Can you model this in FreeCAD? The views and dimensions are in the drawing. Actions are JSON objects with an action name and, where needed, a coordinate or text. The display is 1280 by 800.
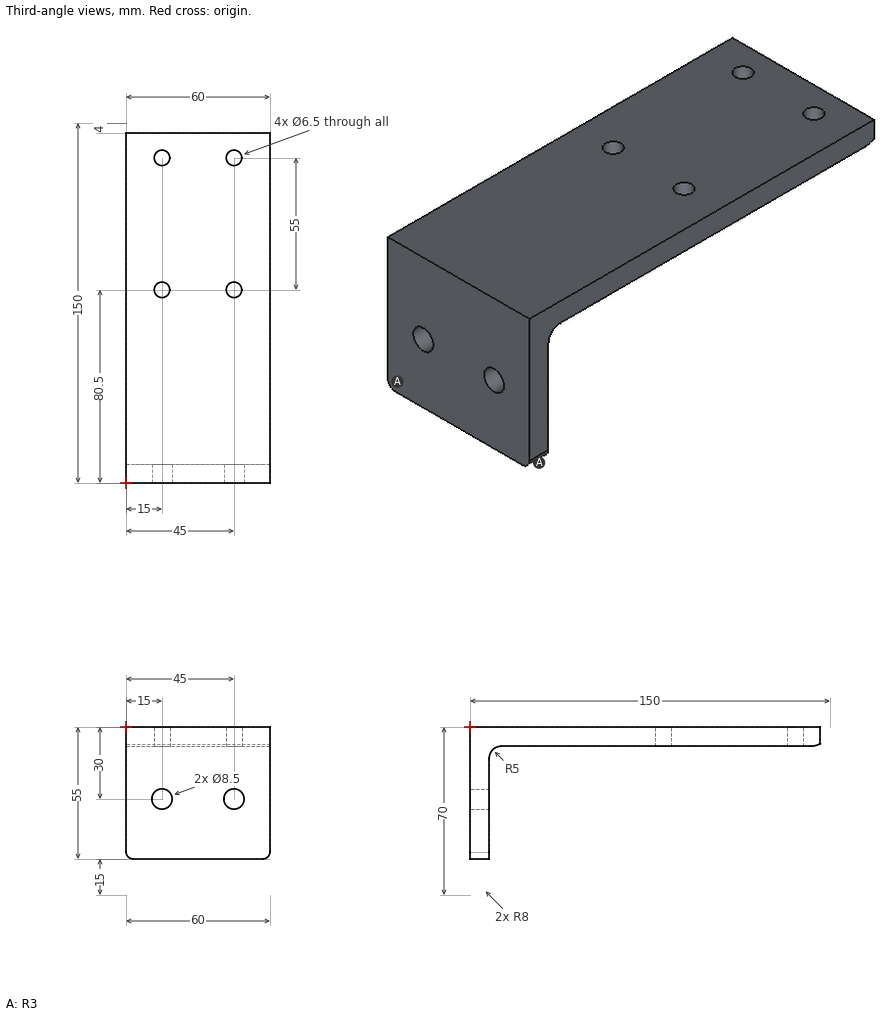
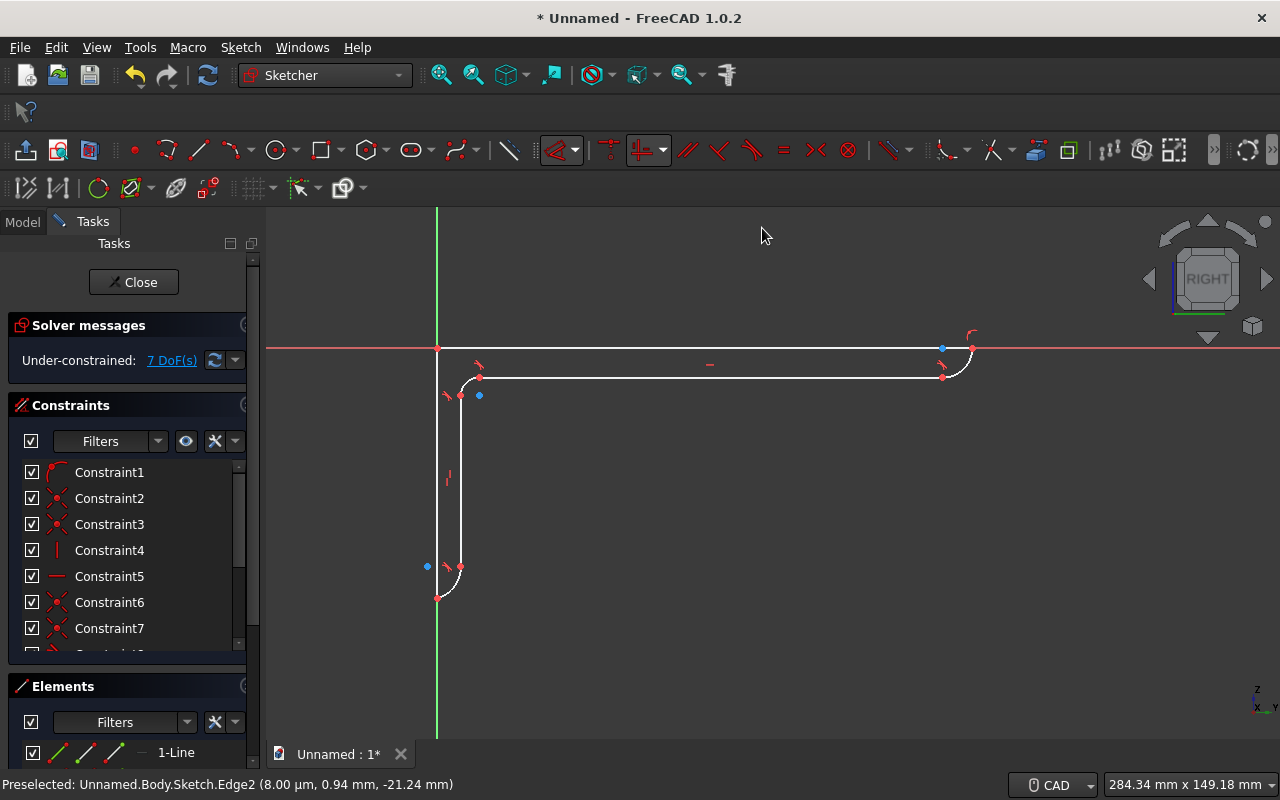
{"action": "scroll", "coordinate": [448, 593], "scroll_direction": "up", "scroll_amount": 2}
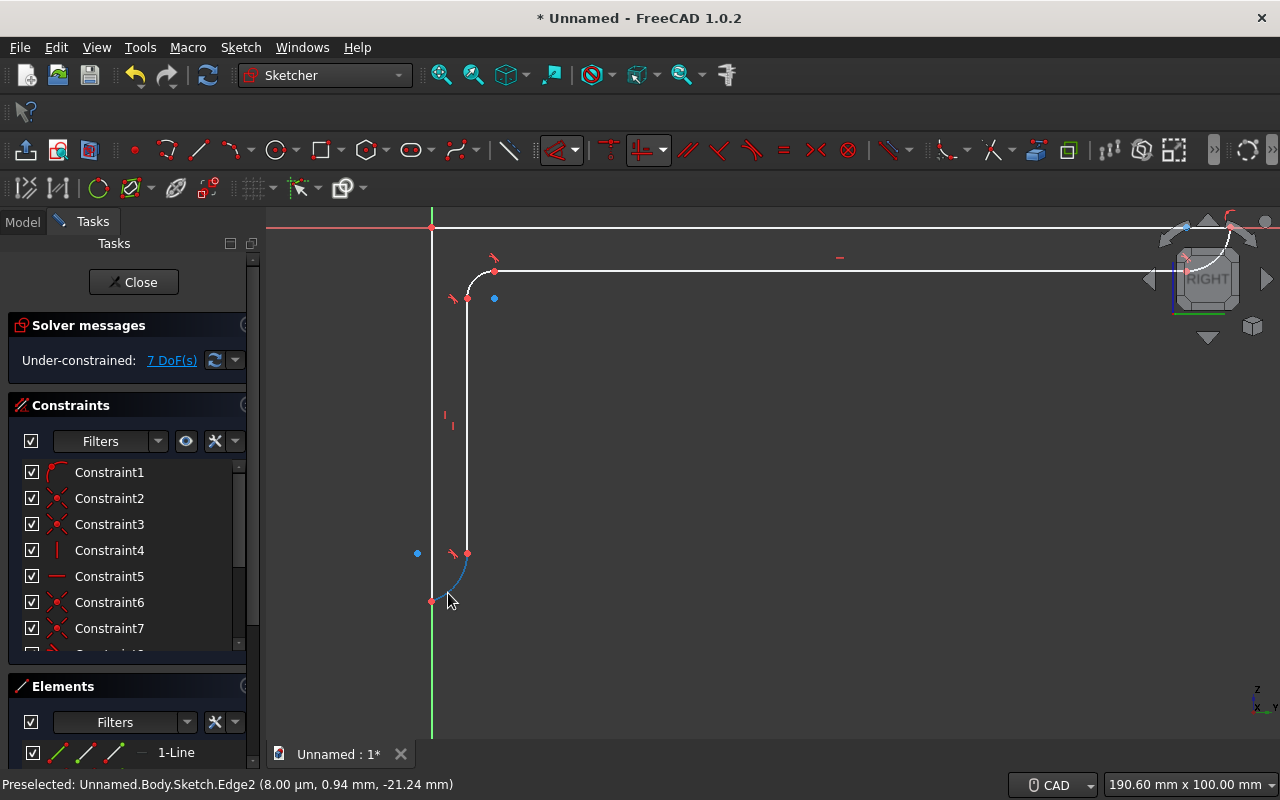
{"action": "left_click", "coordinate": [449, 592]}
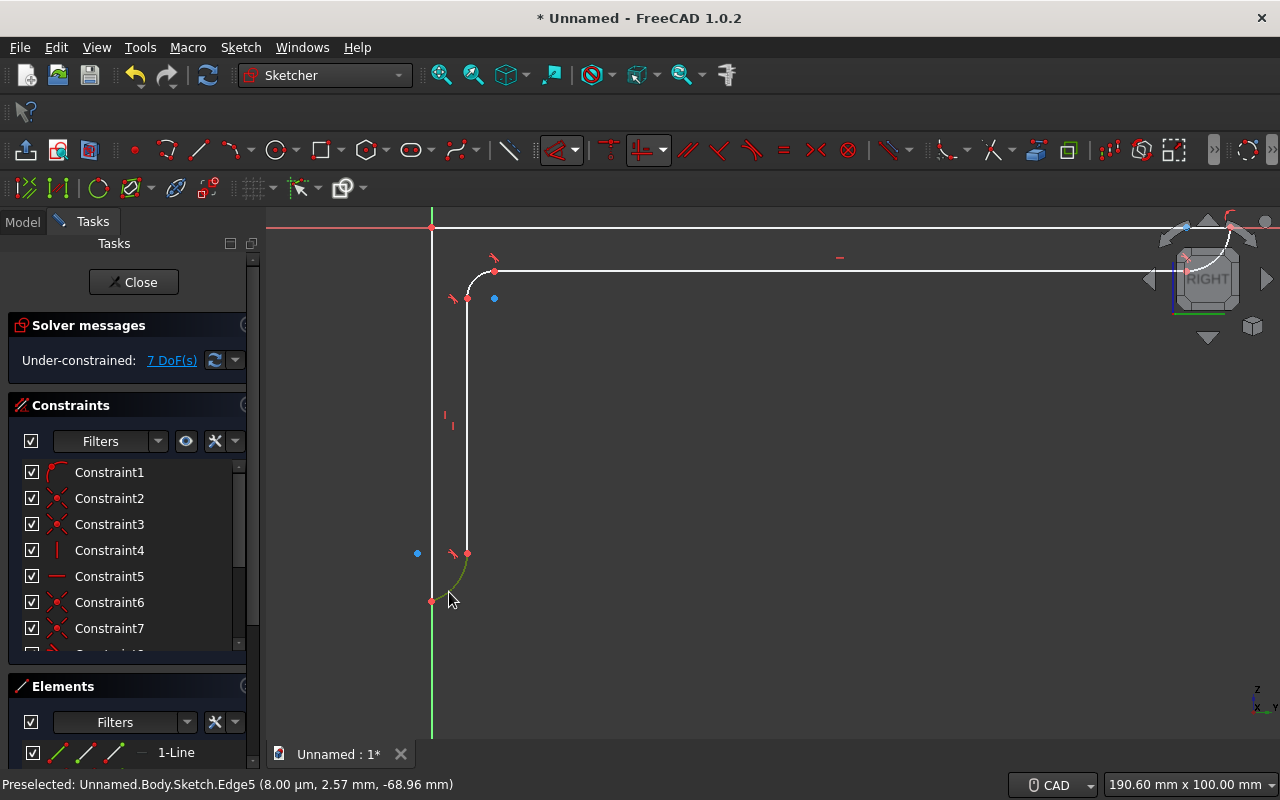
{"action": "scroll", "coordinate": [448, 593], "scroll_direction": "down", "scroll_amount": 2}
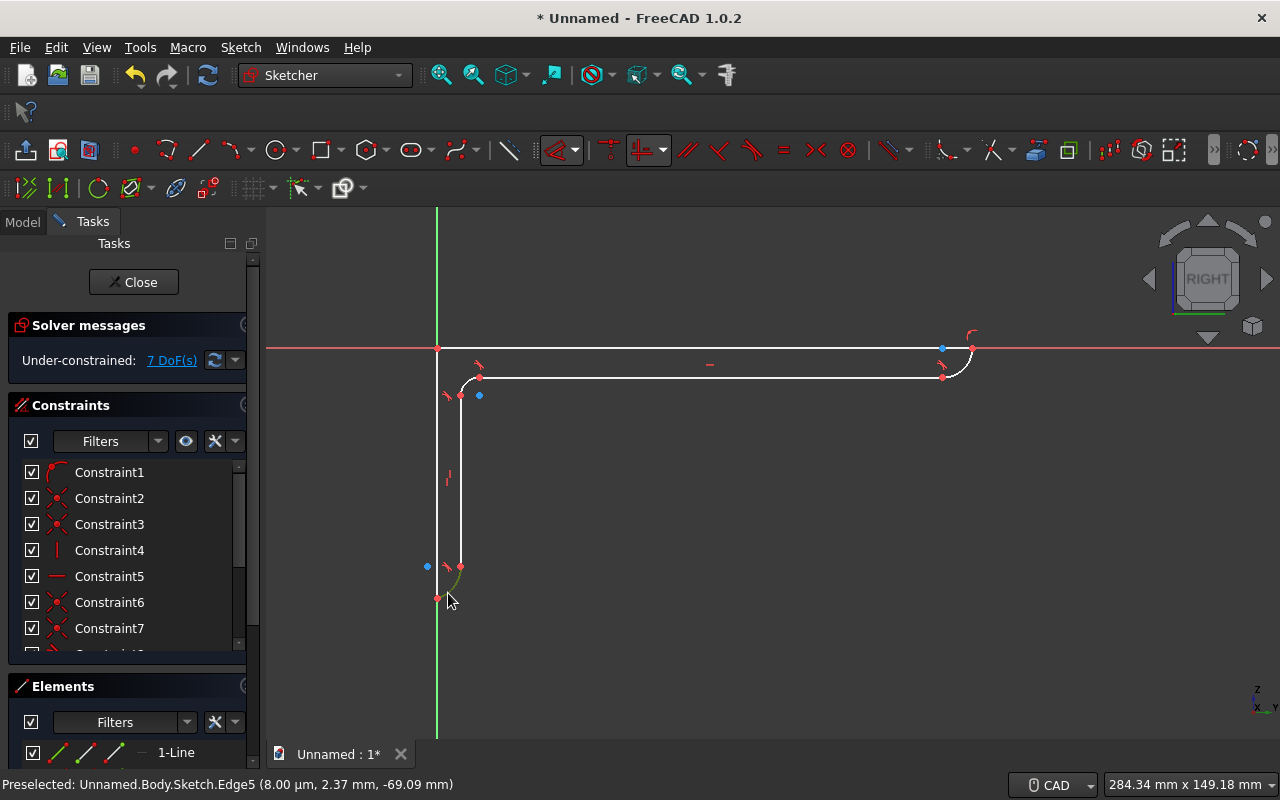
{"action": "left_click", "coordinate": [956, 374]}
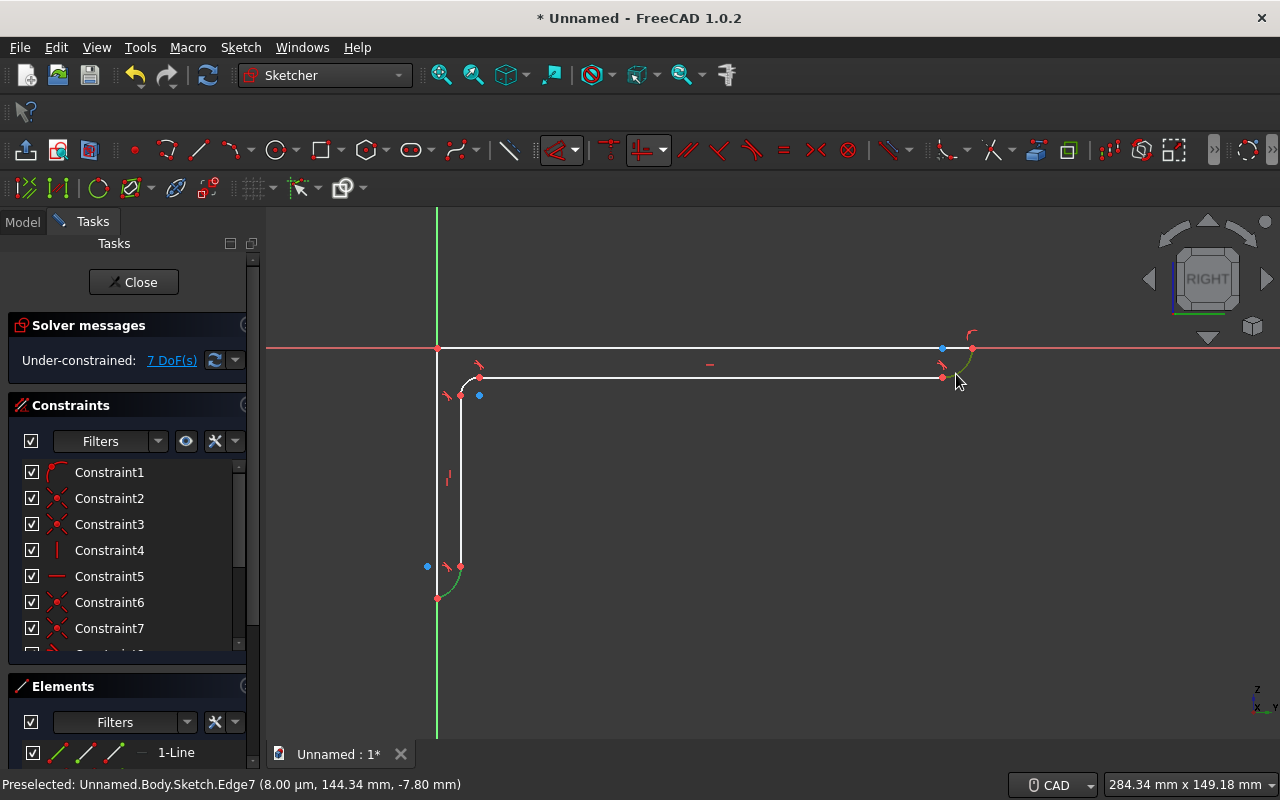
{"action": "key", "text": "e"}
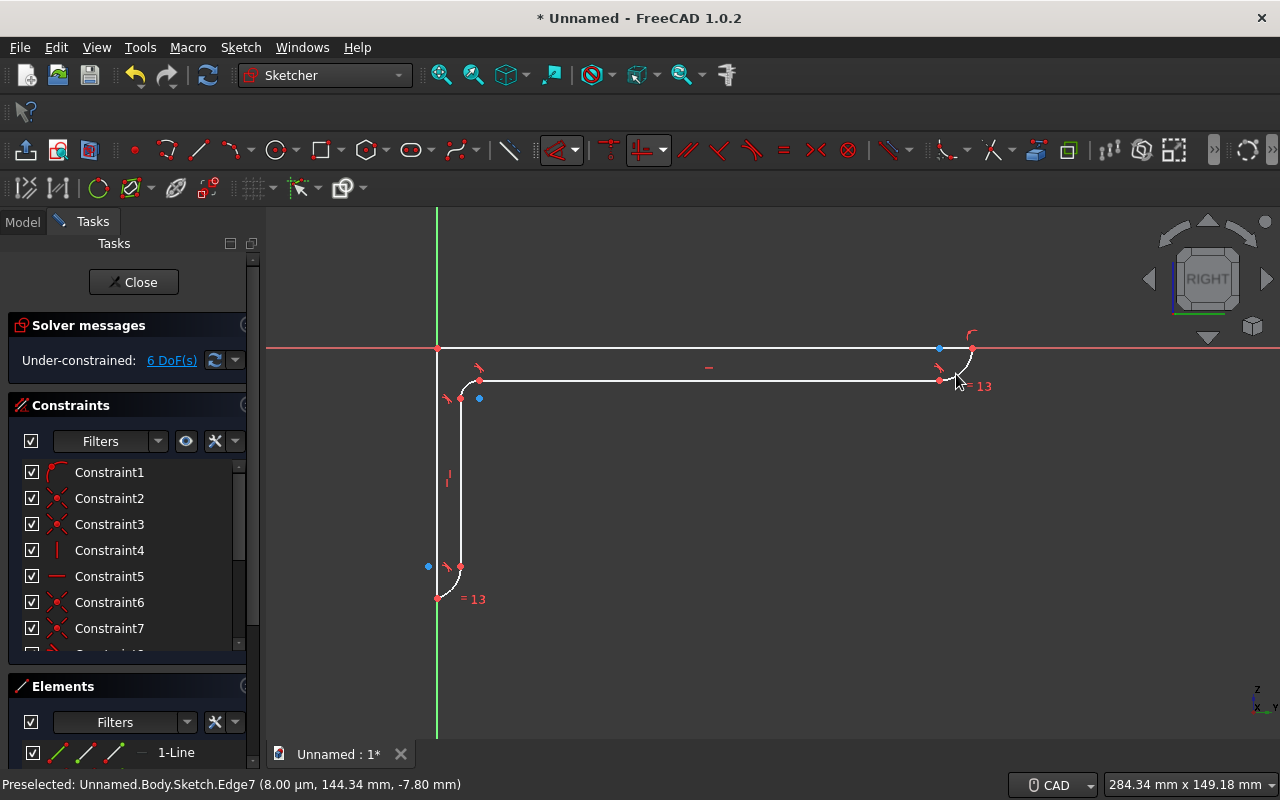
{"action": "left_click", "coordinate": [428, 567]}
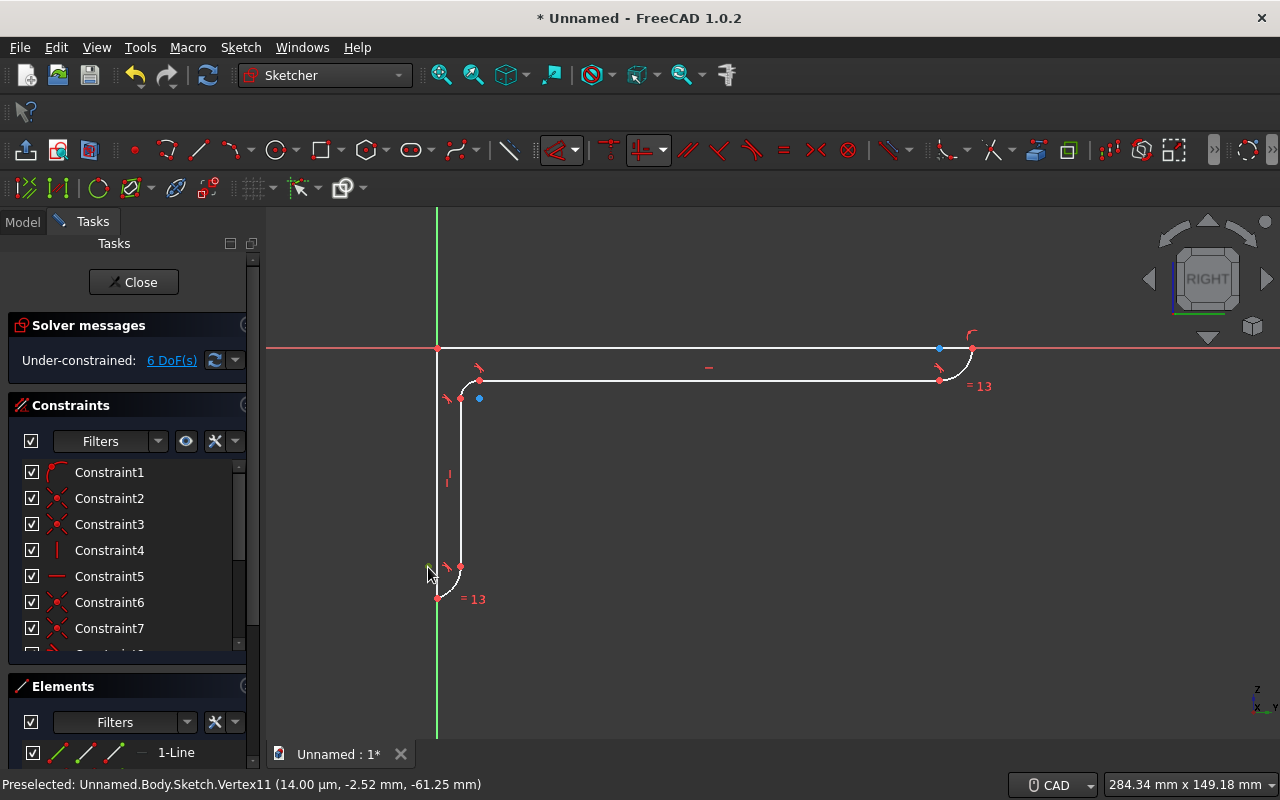
{"action": "left_click", "coordinate": [437, 677]}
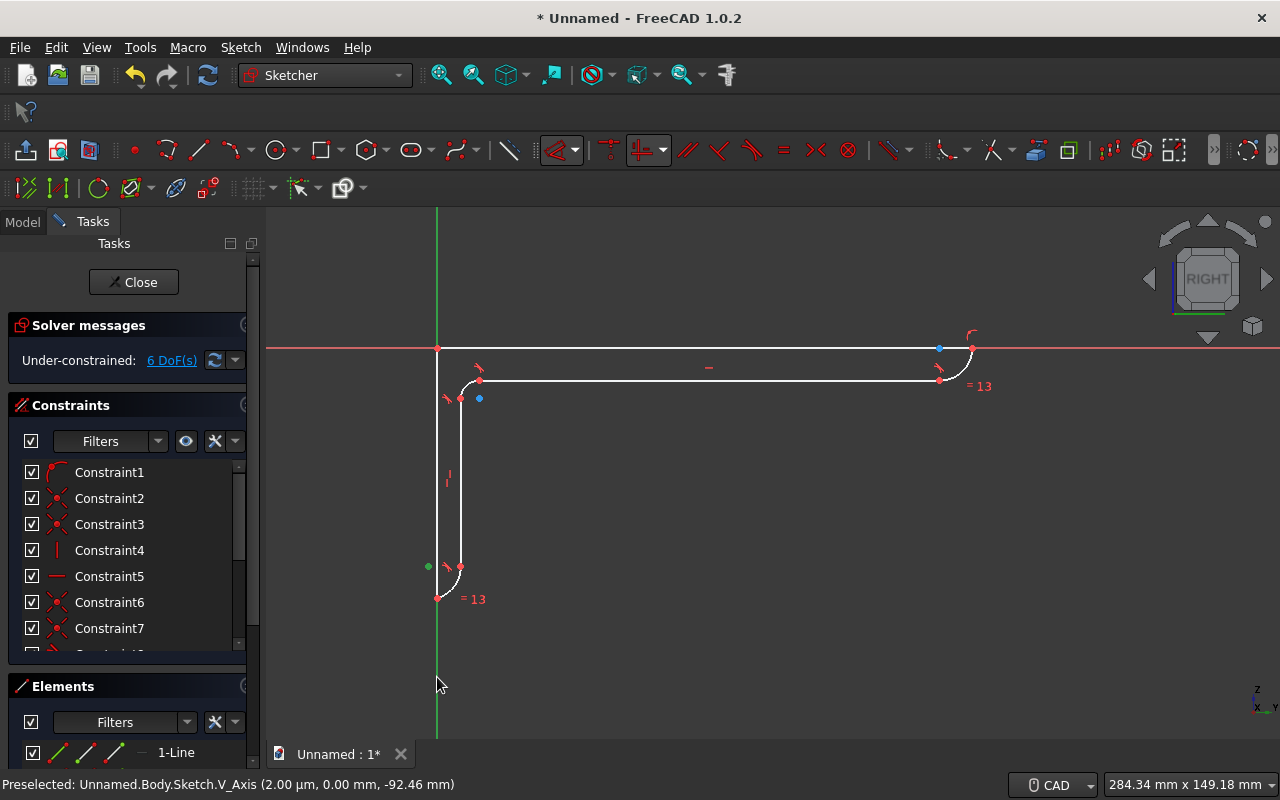
{"action": "key", "text": "c"}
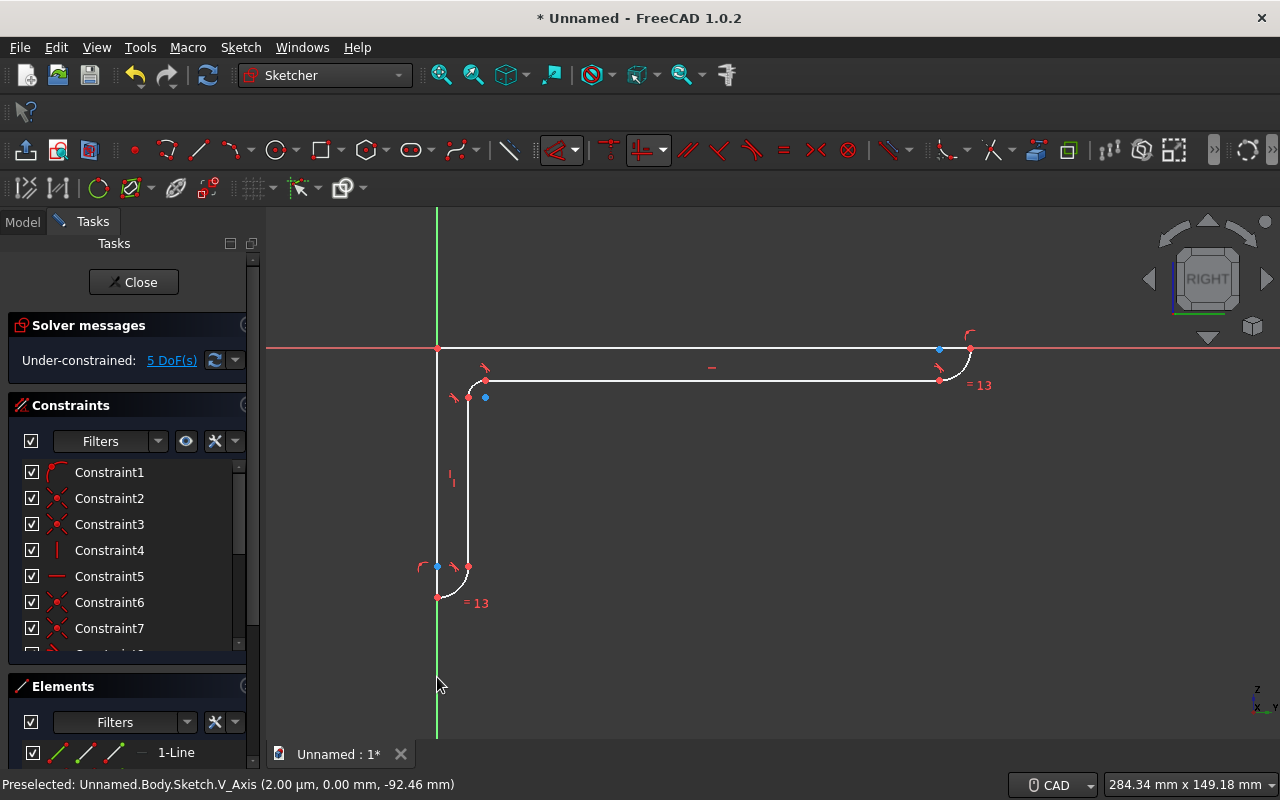
{"action": "left_click", "coordinate": [940, 350]}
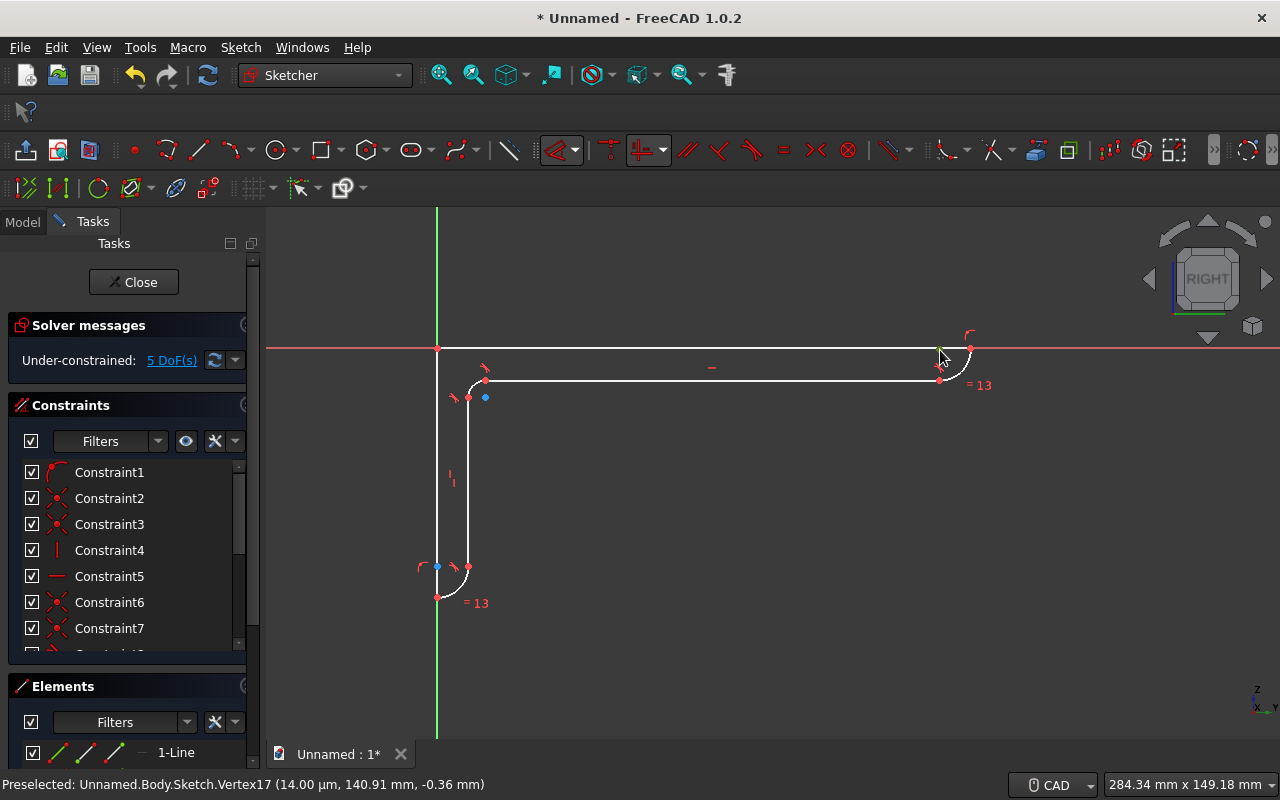
{"action": "left_click", "coordinate": [353, 348]}